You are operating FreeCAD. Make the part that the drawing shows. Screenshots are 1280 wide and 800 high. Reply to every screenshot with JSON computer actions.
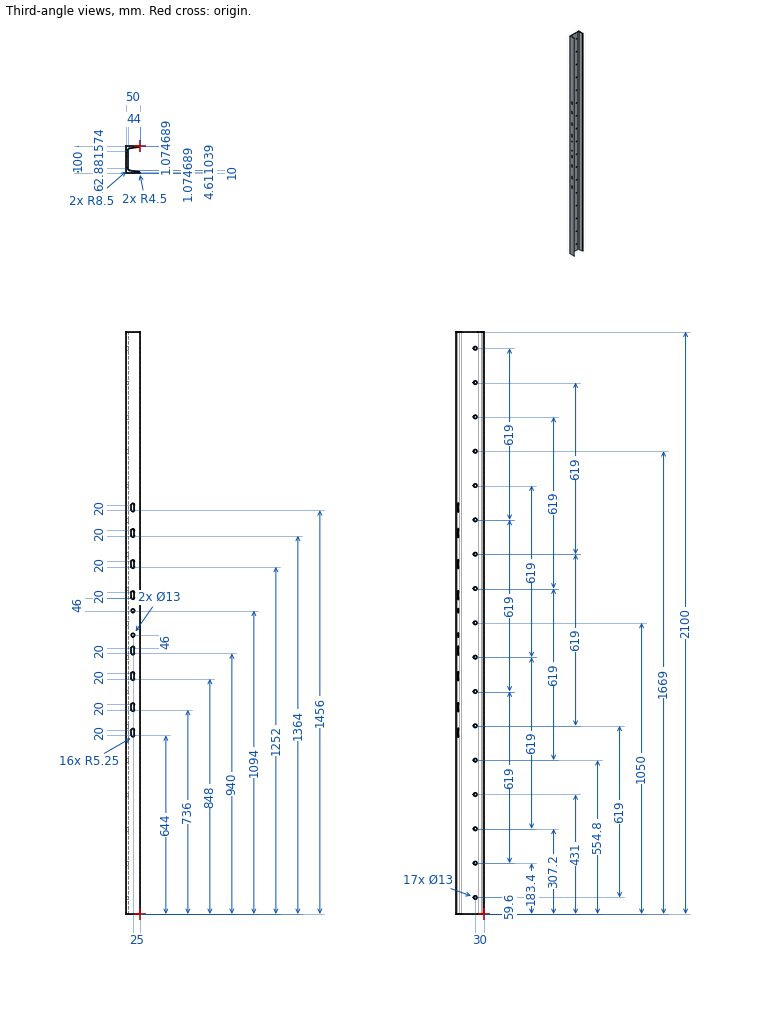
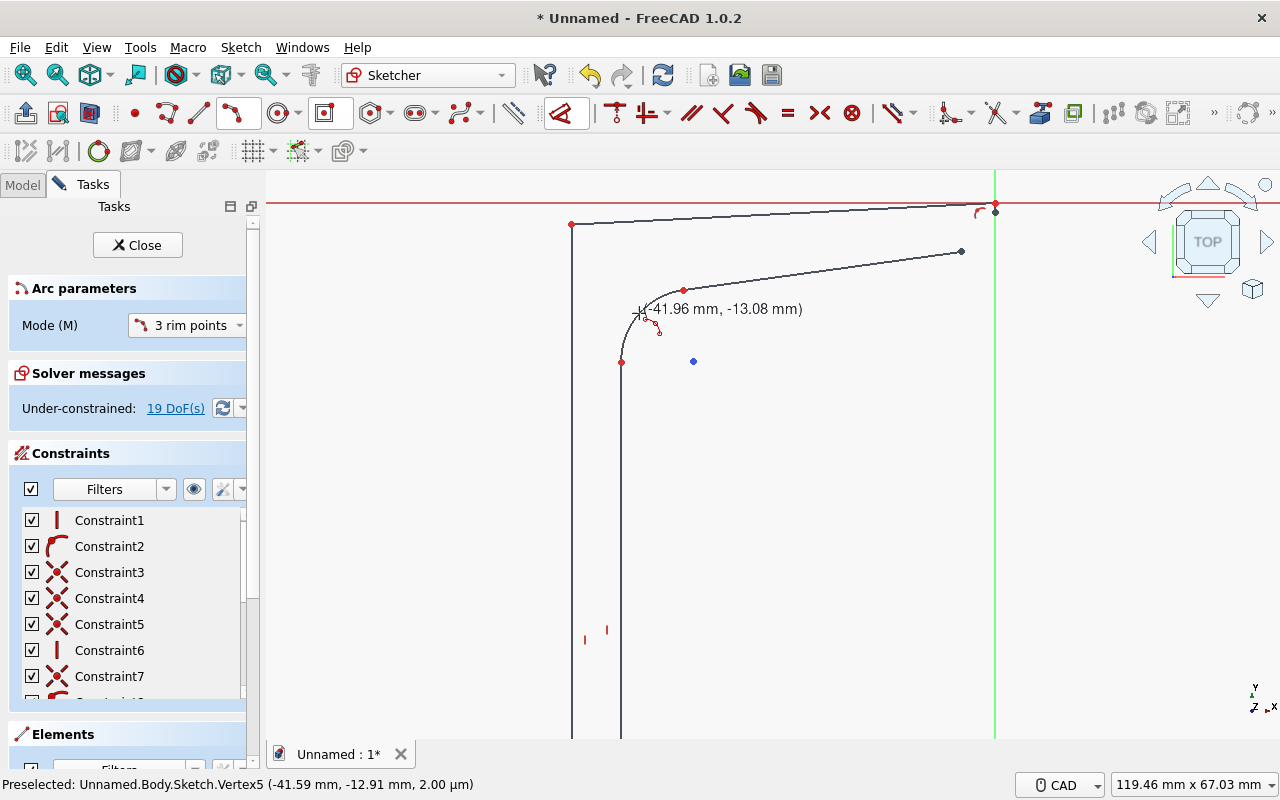
{"action": "left_click", "coordinate": [962, 252]}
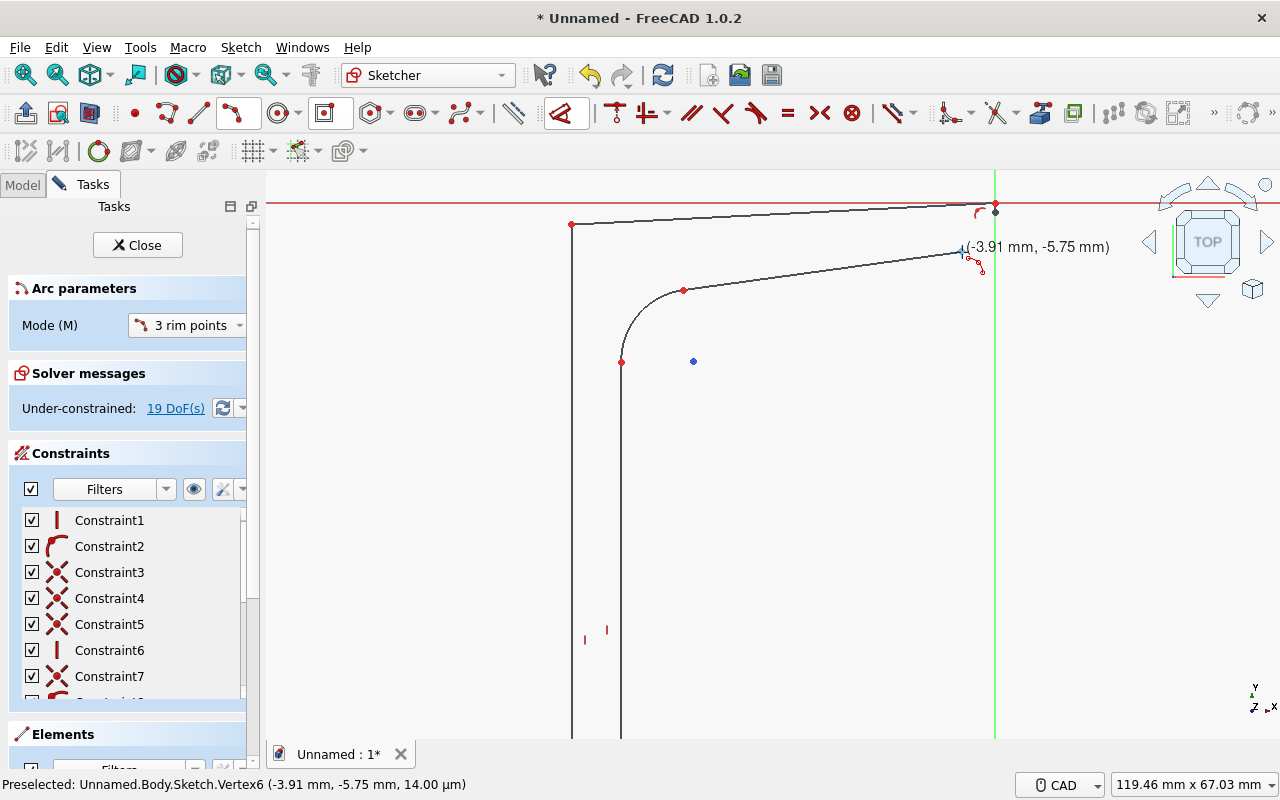
{"action": "scroll", "coordinate": [995, 212], "scroll_direction": "up", "scroll_amount": 7}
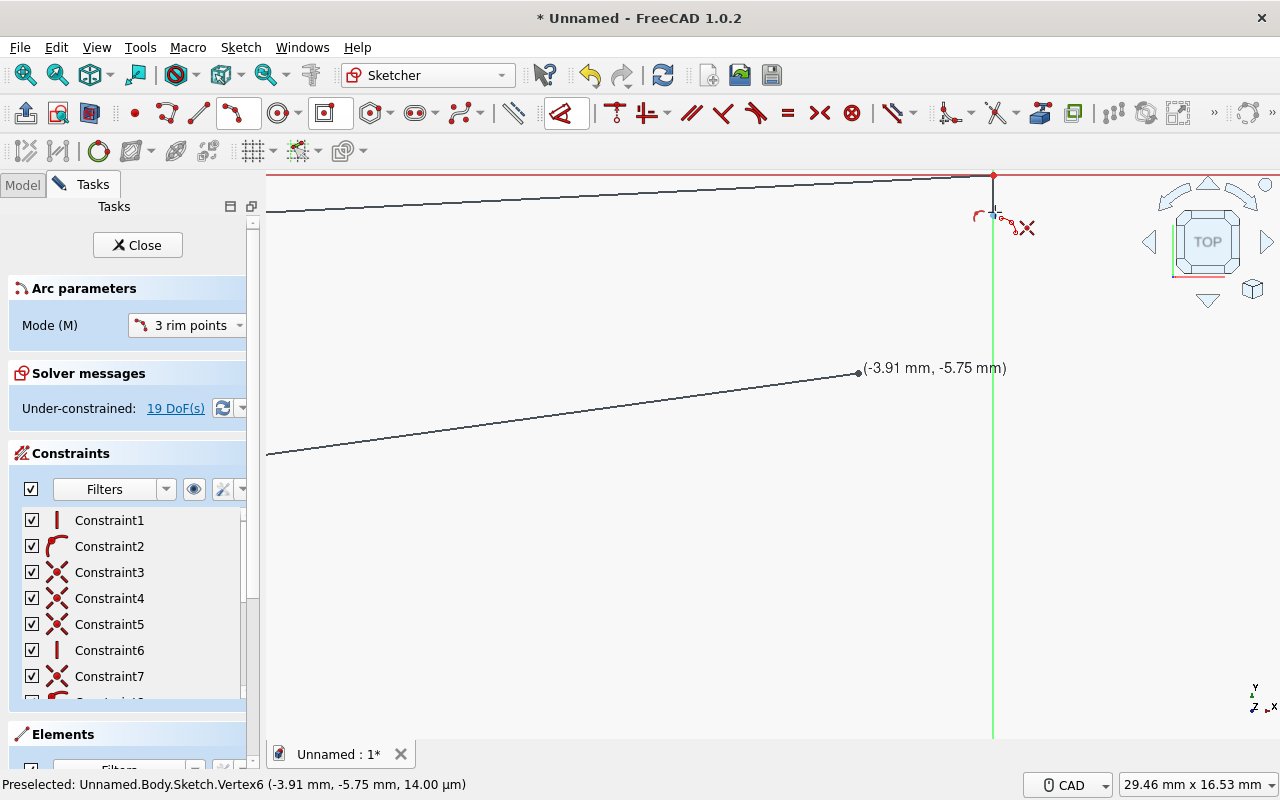
{"action": "left_click", "coordinate": [993, 215]}
{"action": "left_click", "coordinate": [956, 314]}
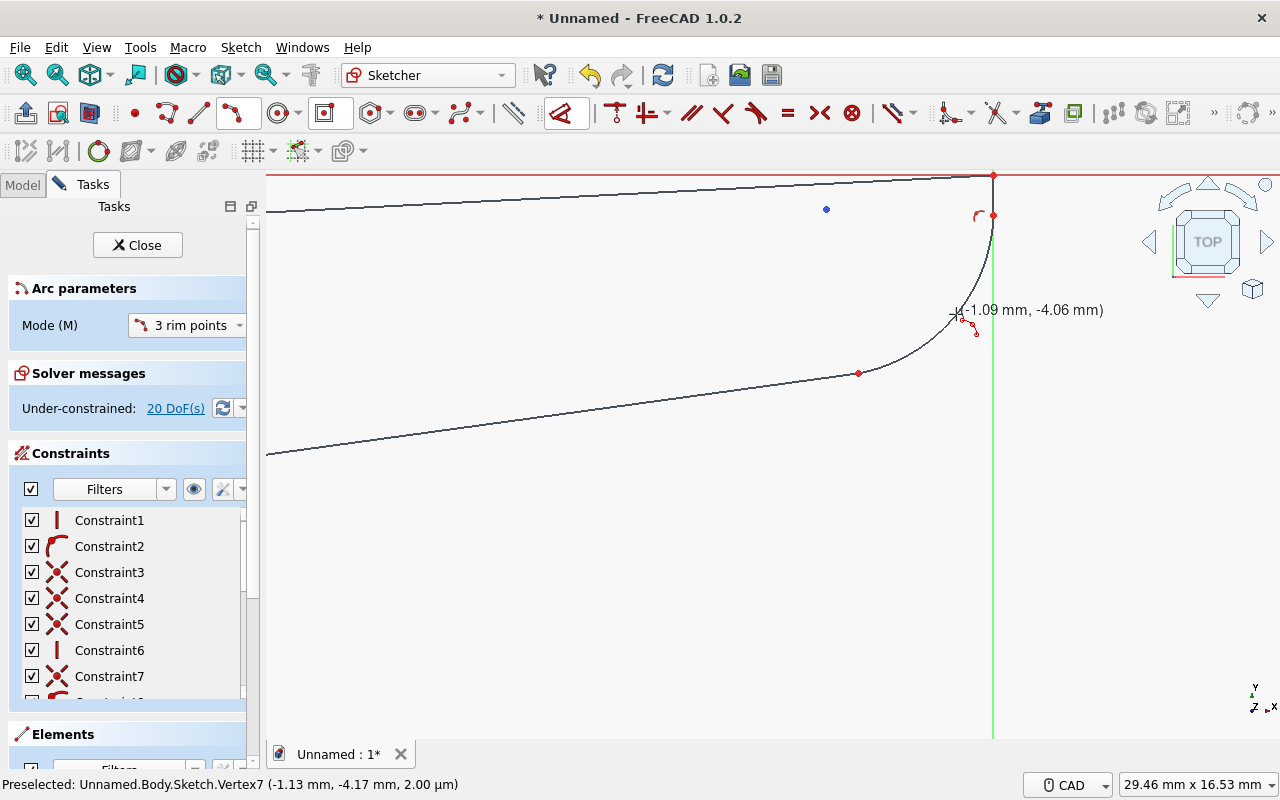
{"action": "scroll", "coordinate": [776, 275], "scroll_direction": "down", "scroll_amount": 11}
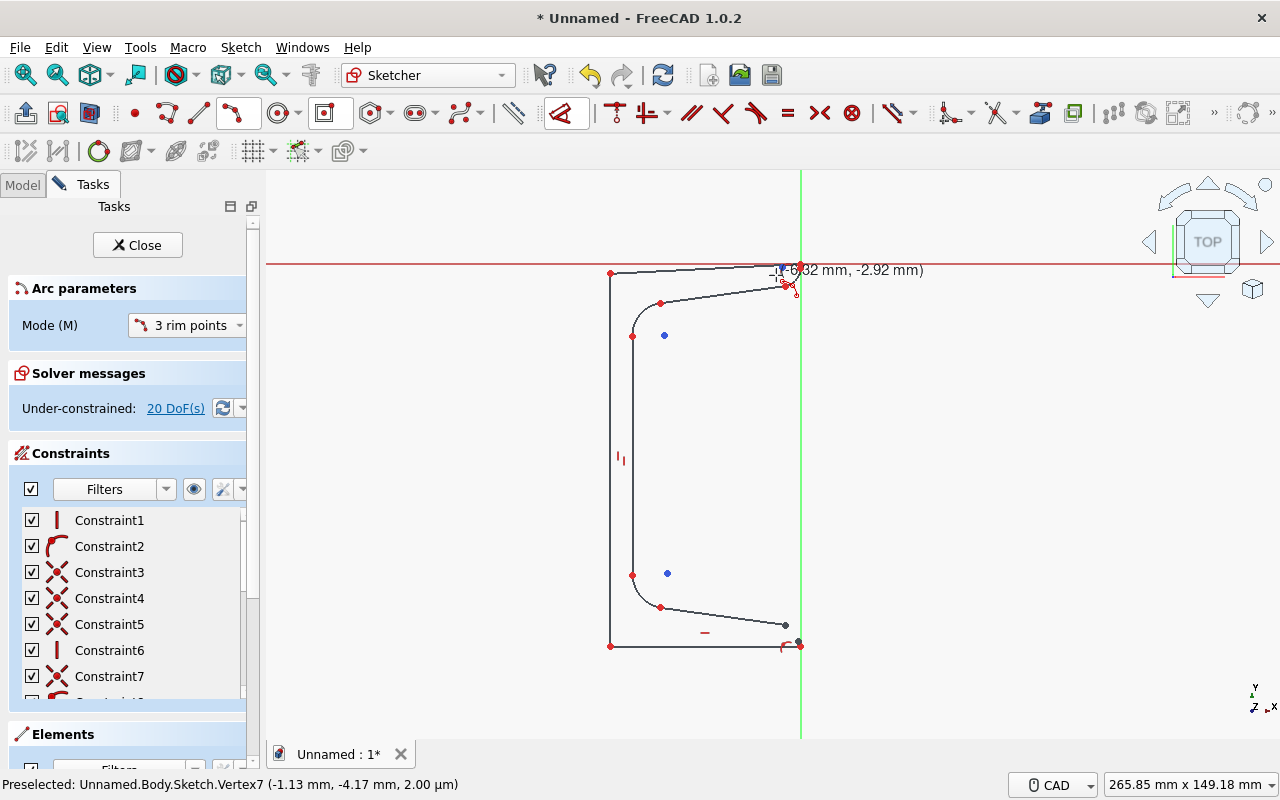
{"action": "scroll", "coordinate": [801, 641], "scroll_direction": "up", "scroll_amount": 11}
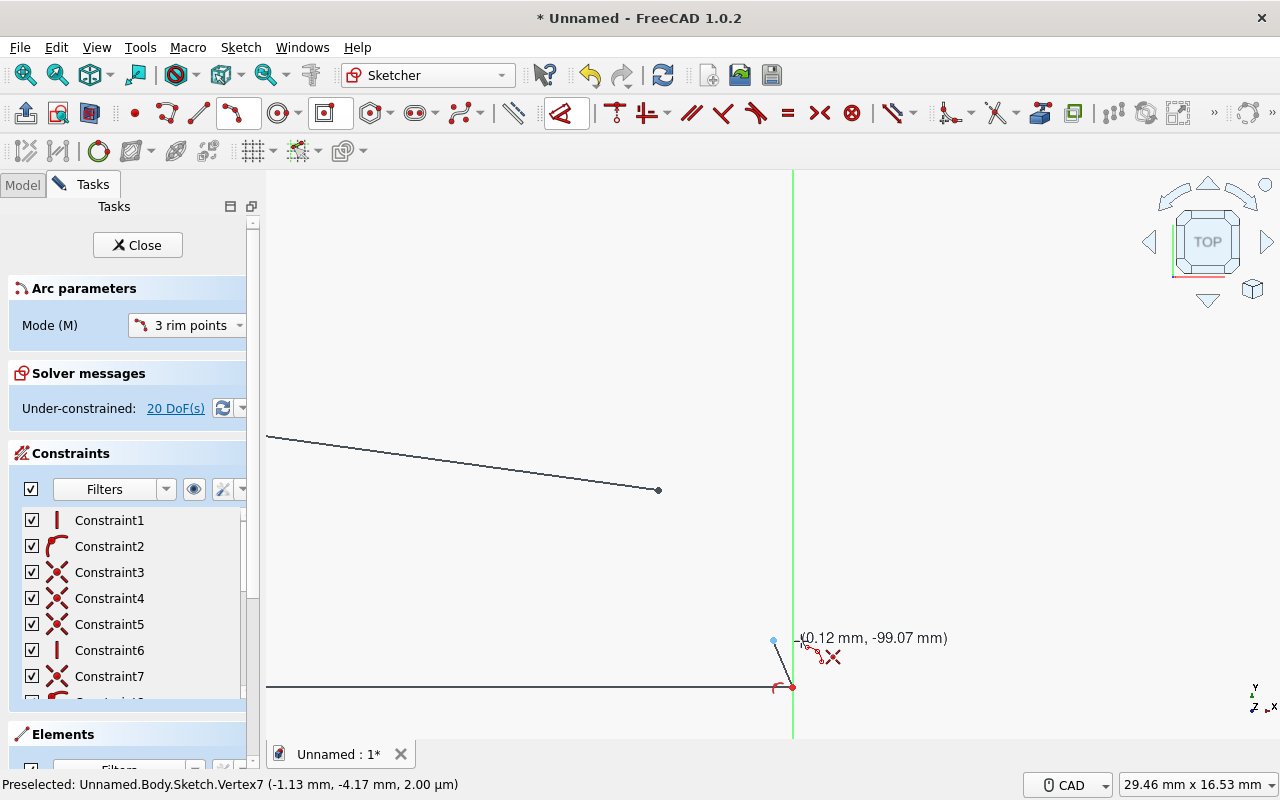
{"action": "left_click", "coordinate": [773, 641]}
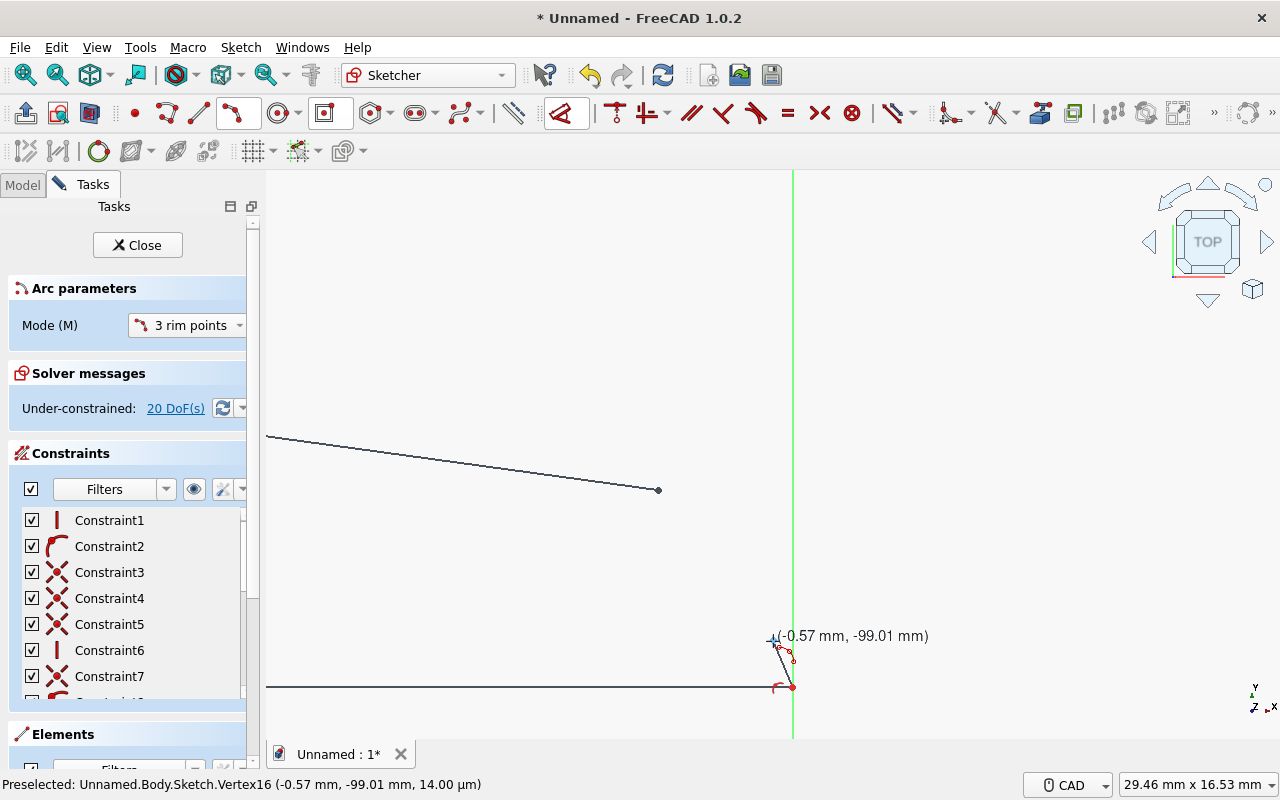
{"action": "scroll", "coordinate": [801, 641], "scroll_direction": "down", "scroll_amount": 11}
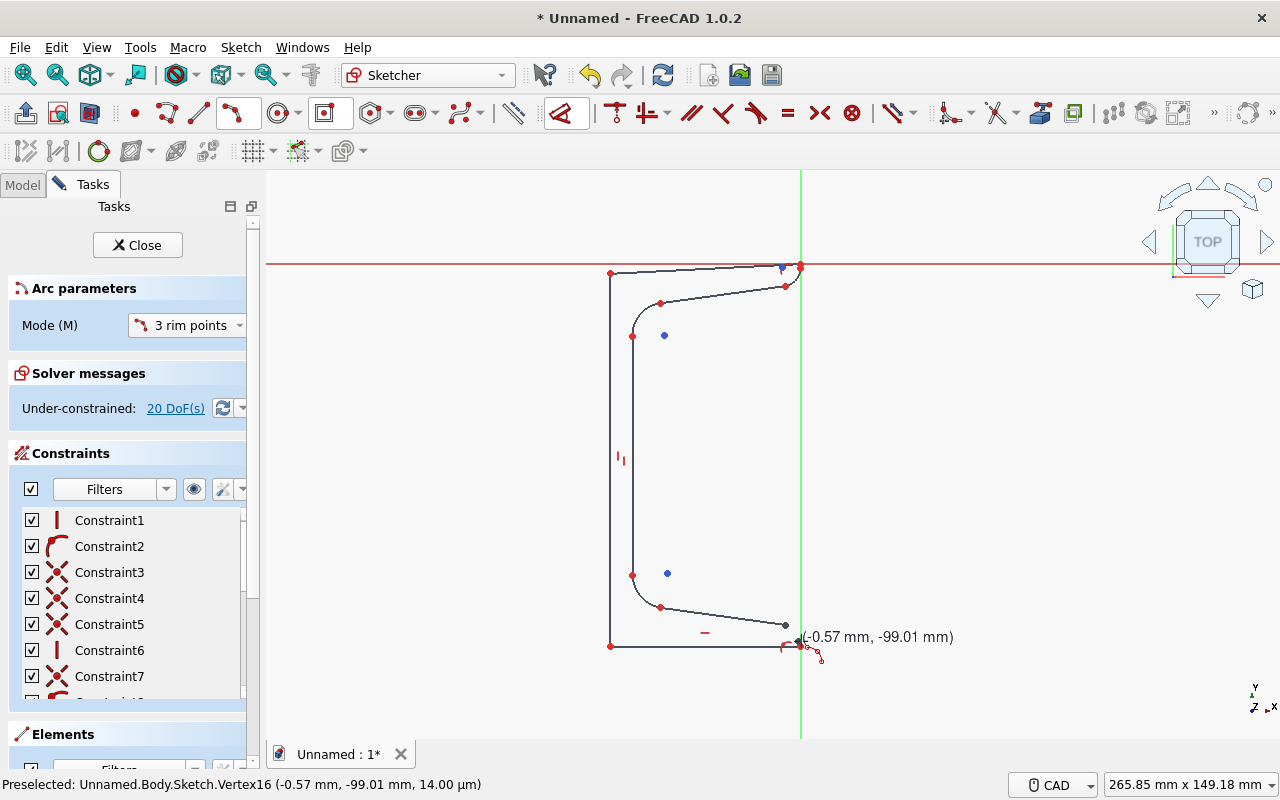
{"action": "left_click", "coordinate": [786, 625]}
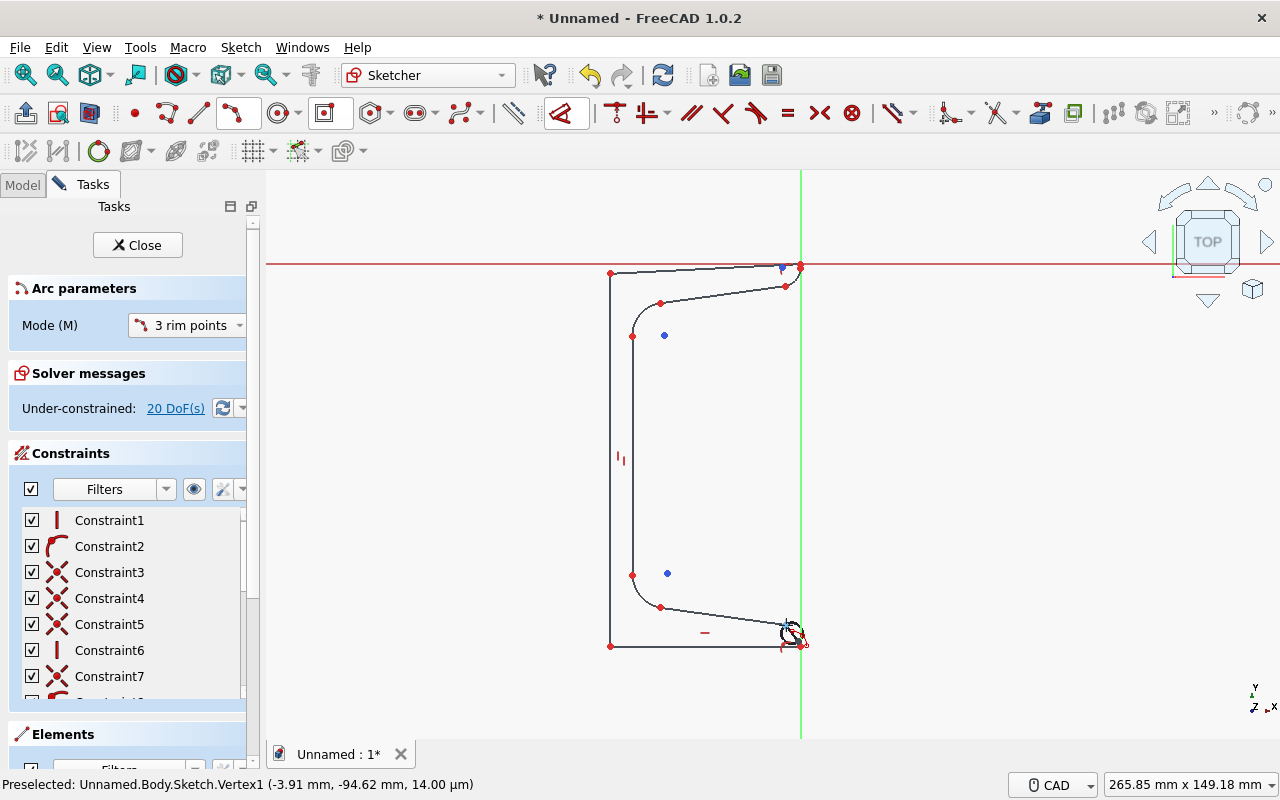
{"action": "scroll", "coordinate": [796, 630], "scroll_direction": "up", "scroll_amount": 7}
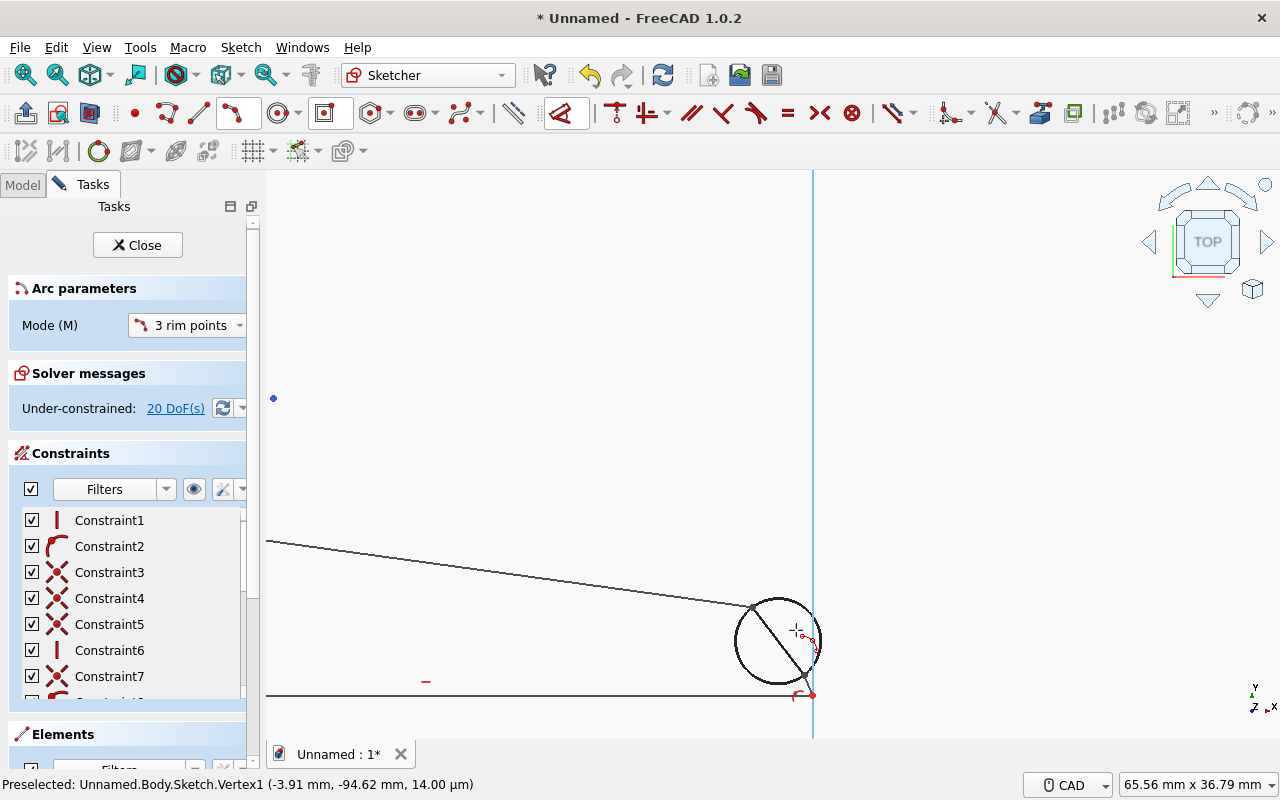
{"action": "left_click", "coordinate": [796, 628]}
{"action": "key", "text": "Escape"}